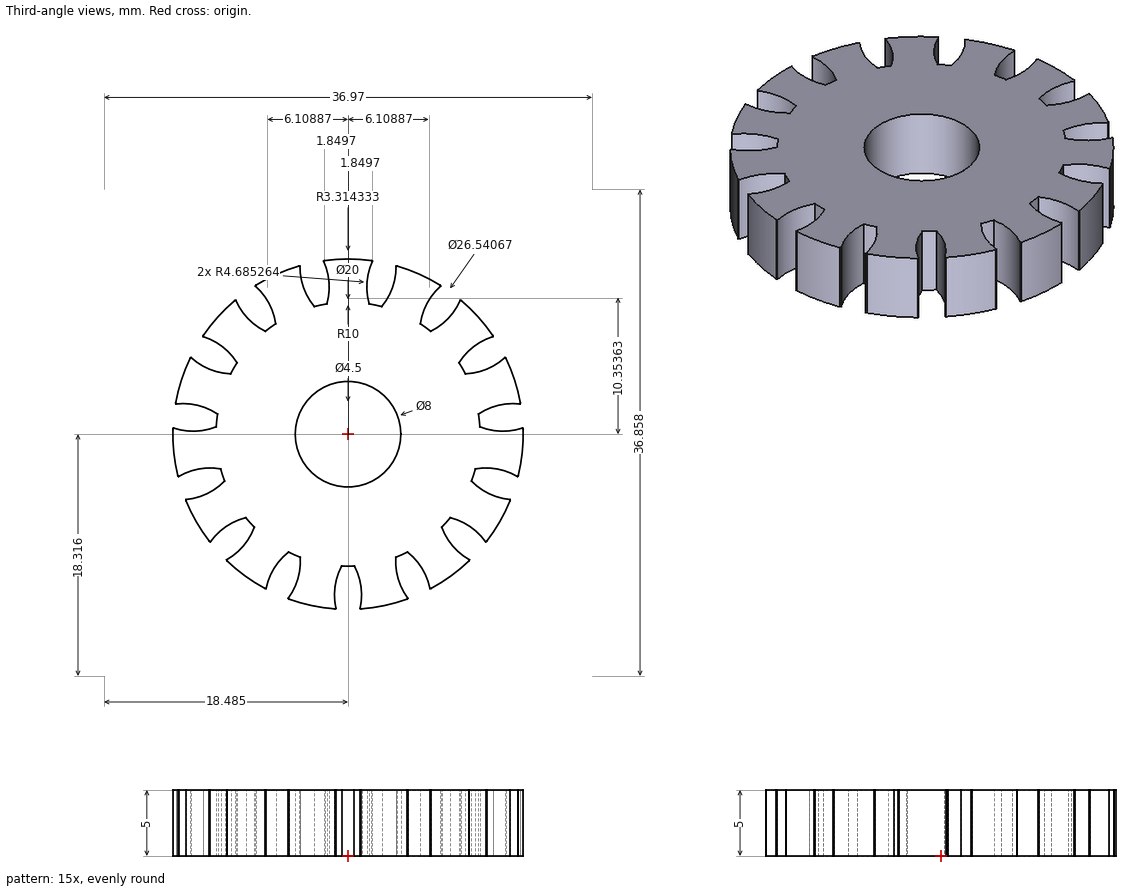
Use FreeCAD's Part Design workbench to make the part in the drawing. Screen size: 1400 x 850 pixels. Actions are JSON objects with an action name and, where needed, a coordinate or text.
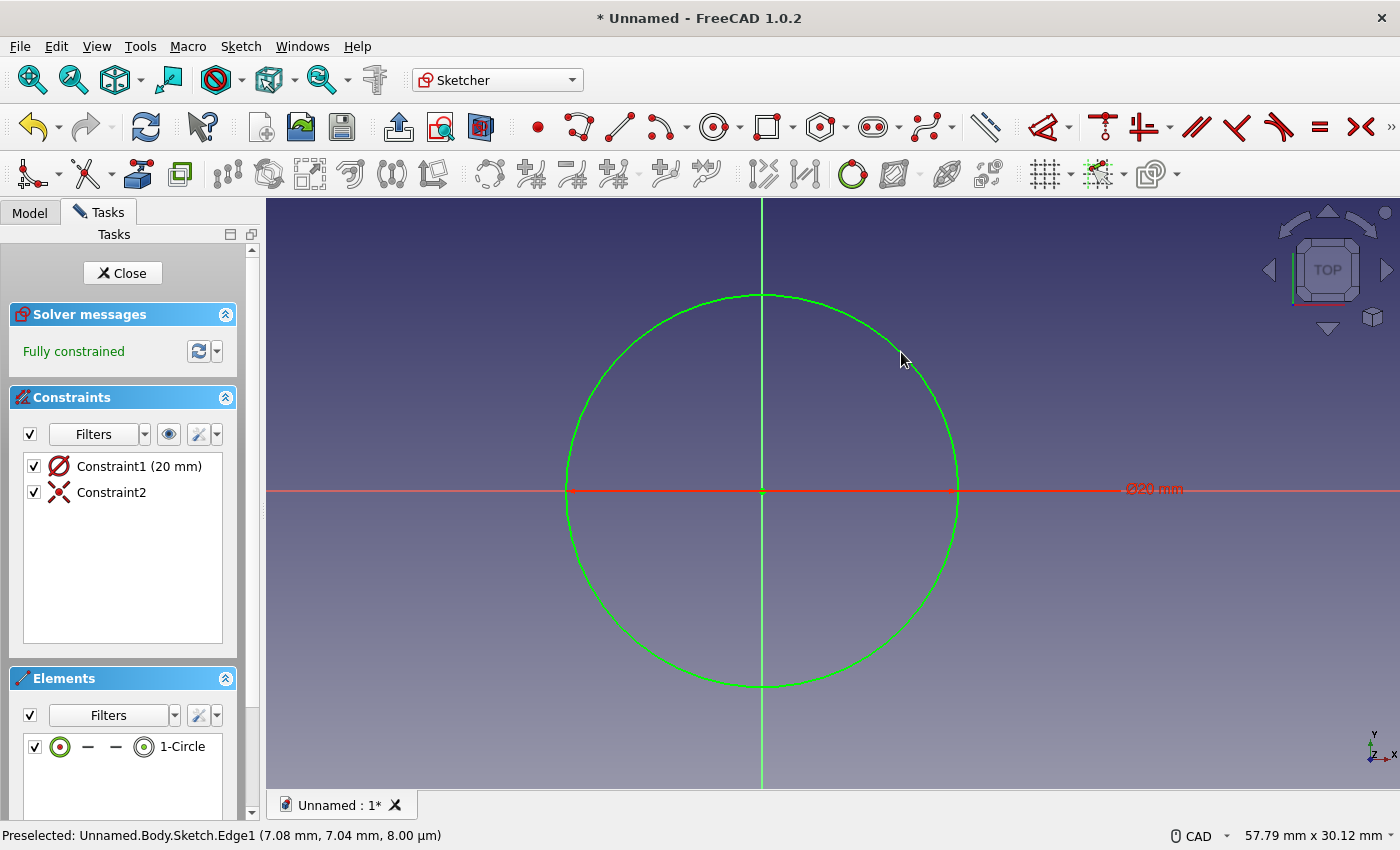
{"action": "left_click", "coordinate": [123, 273]}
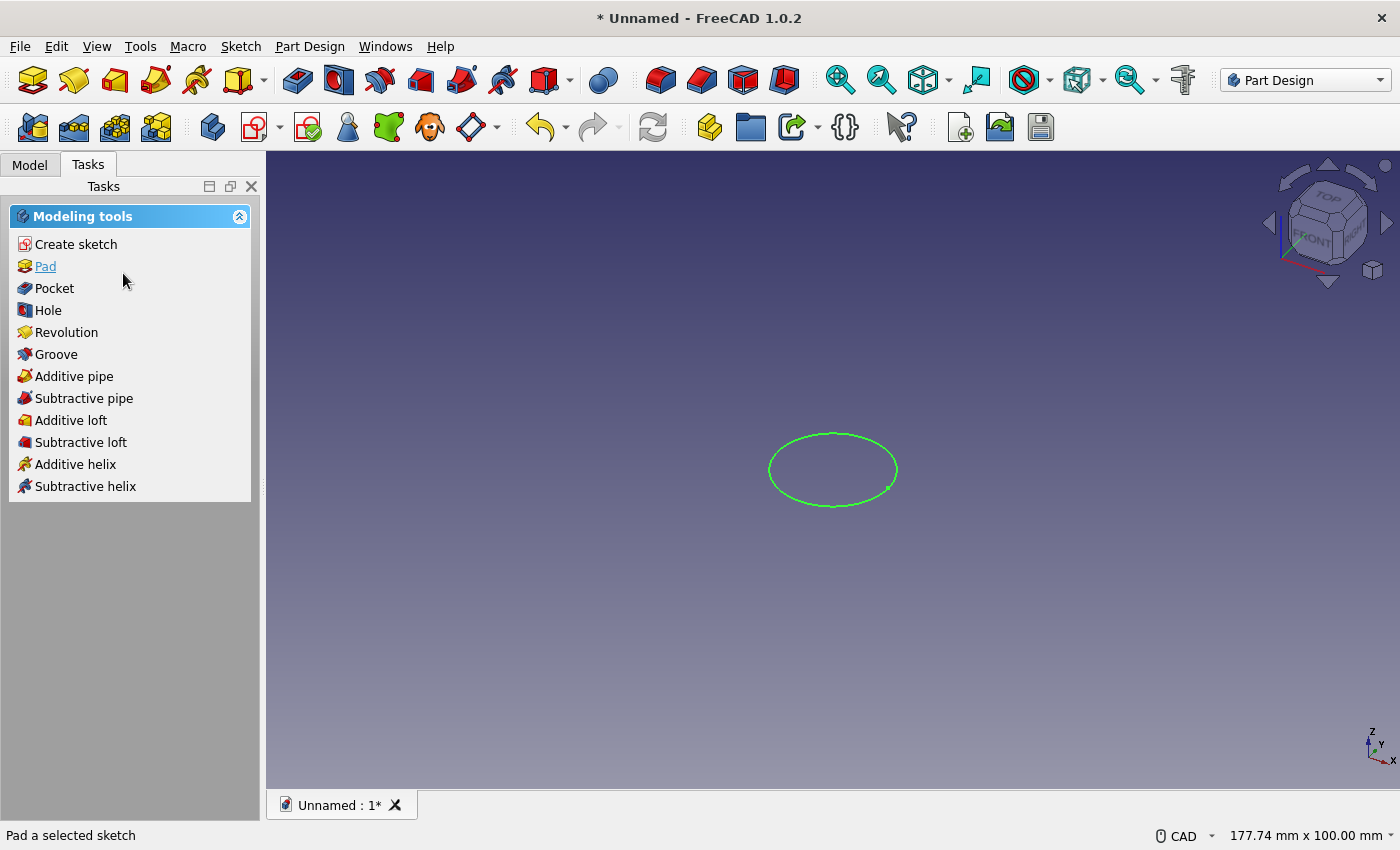
{"action": "left_click", "coordinate": [33, 80]}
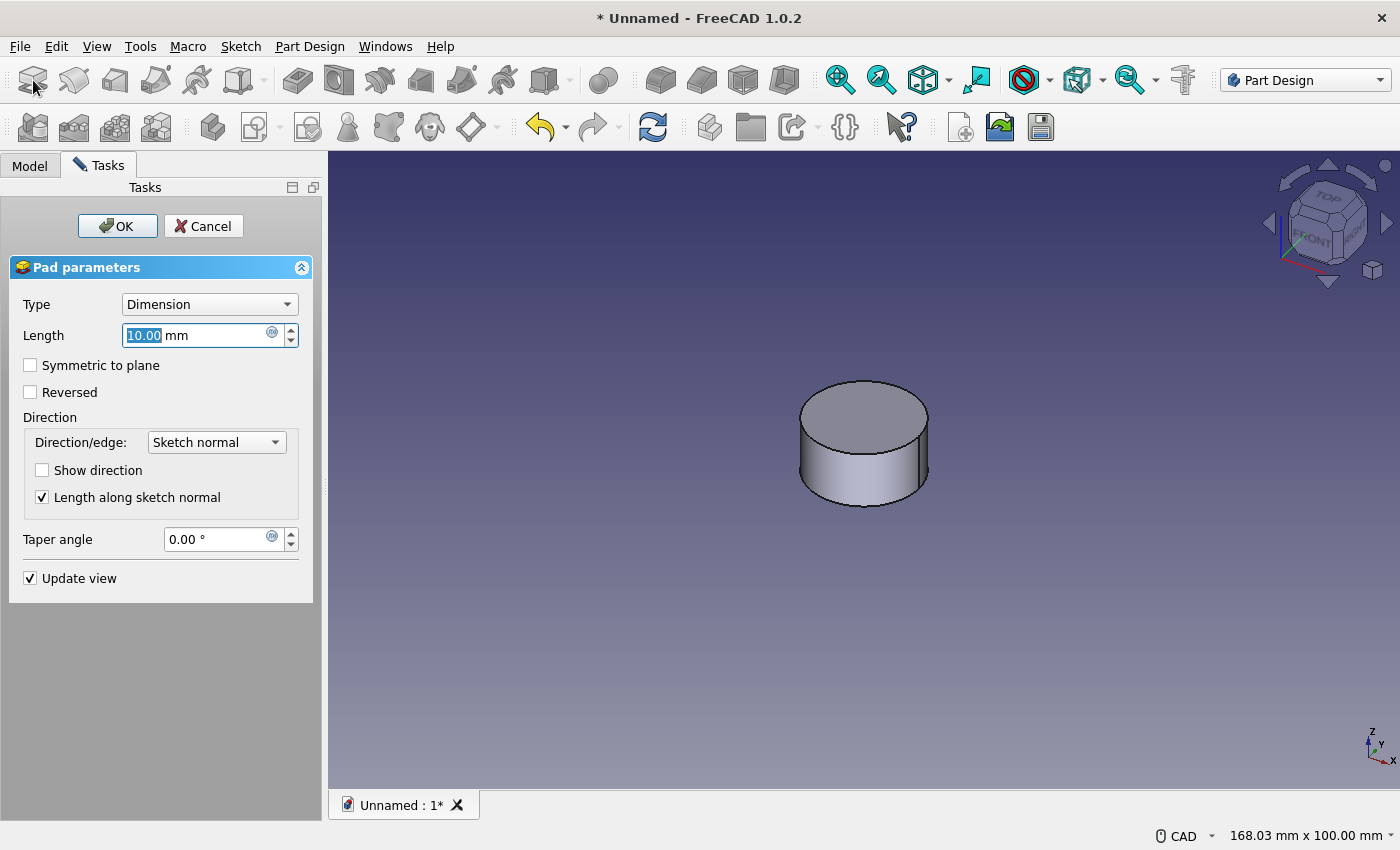
{"action": "type", "text": "5"}
{"action": "key", "text": "Tab"}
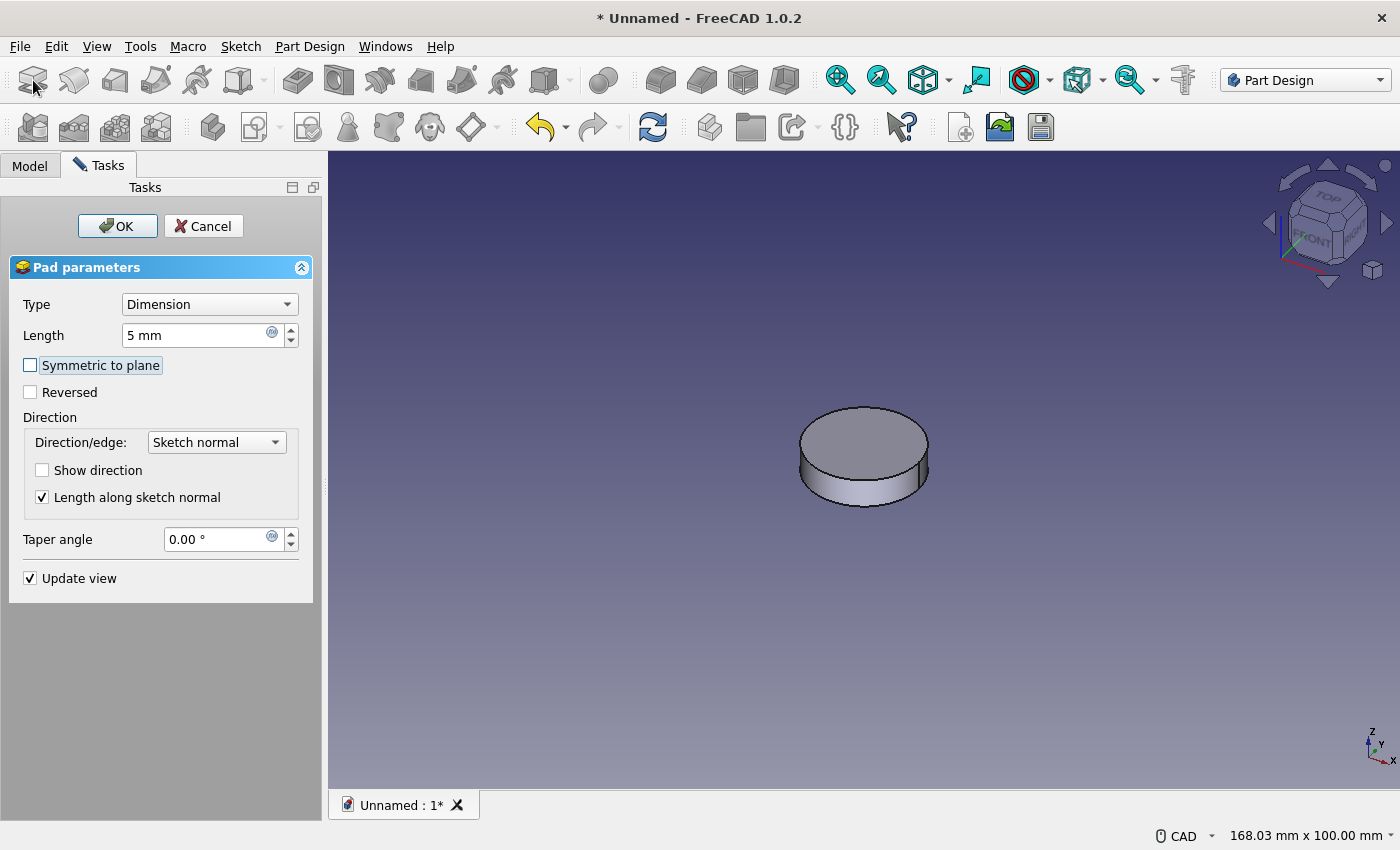
{"action": "left_click", "coordinate": [118, 226]}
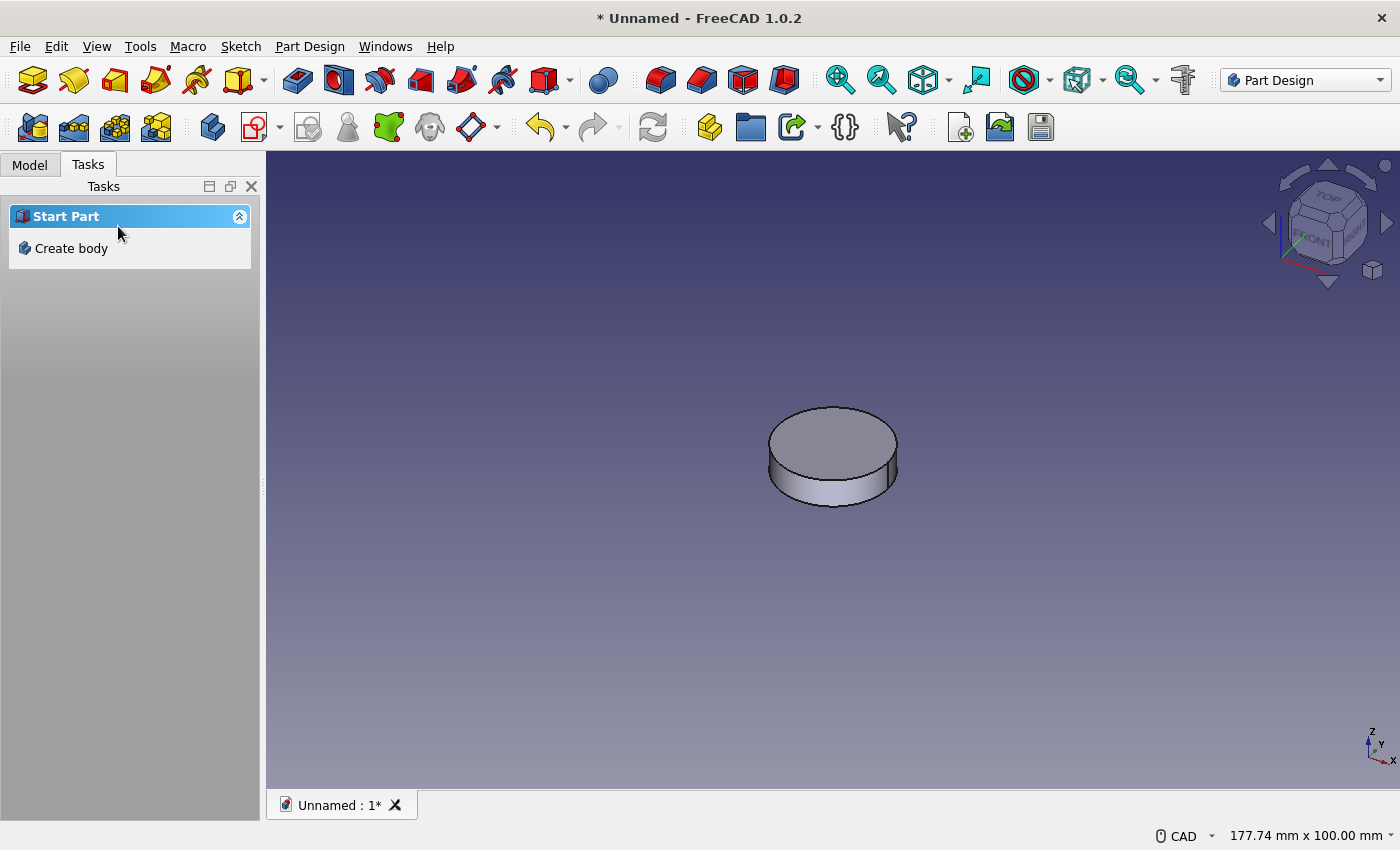
{"action": "key", "text": "v f"}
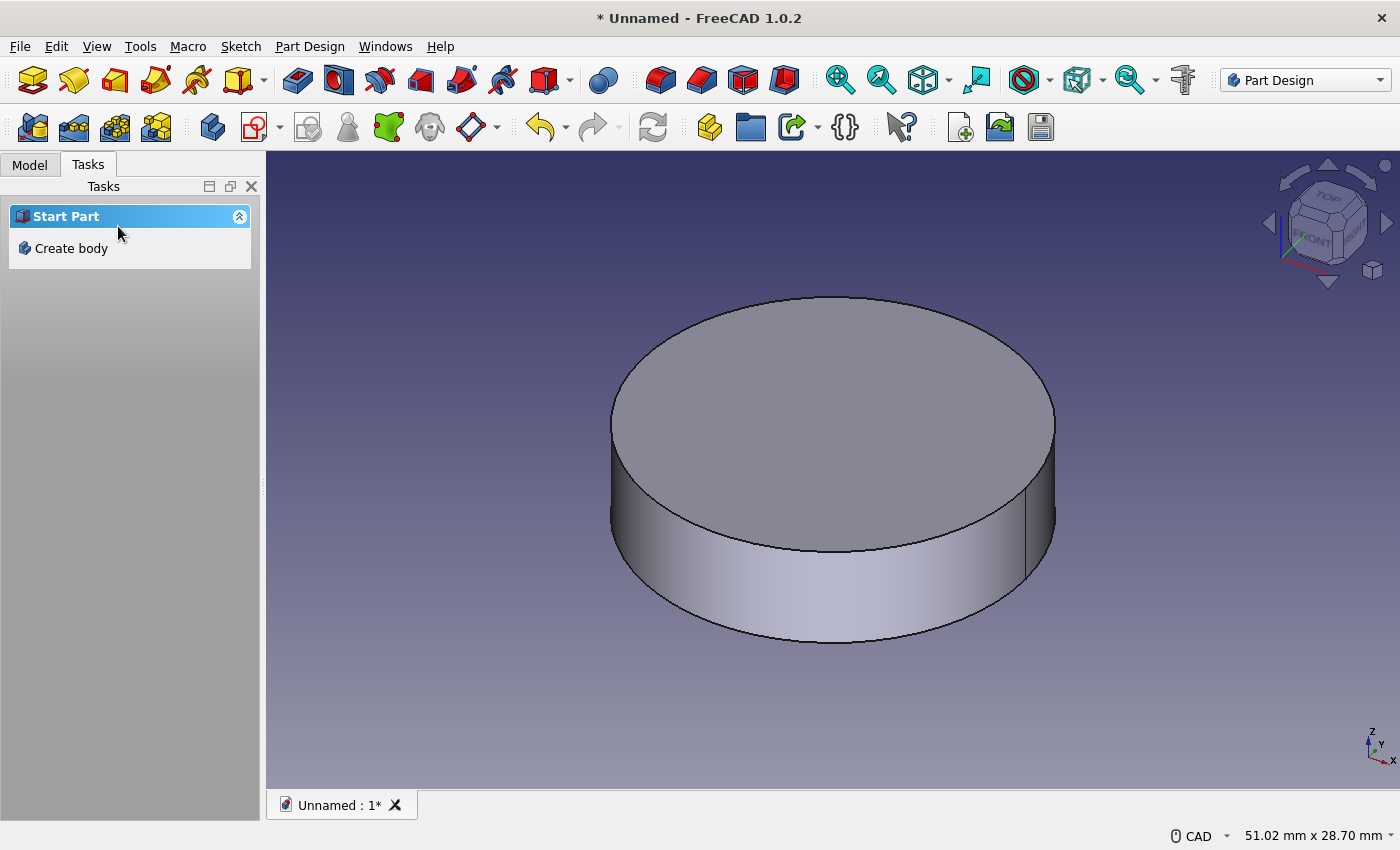
{"action": "left_click", "coordinate": [254, 128]}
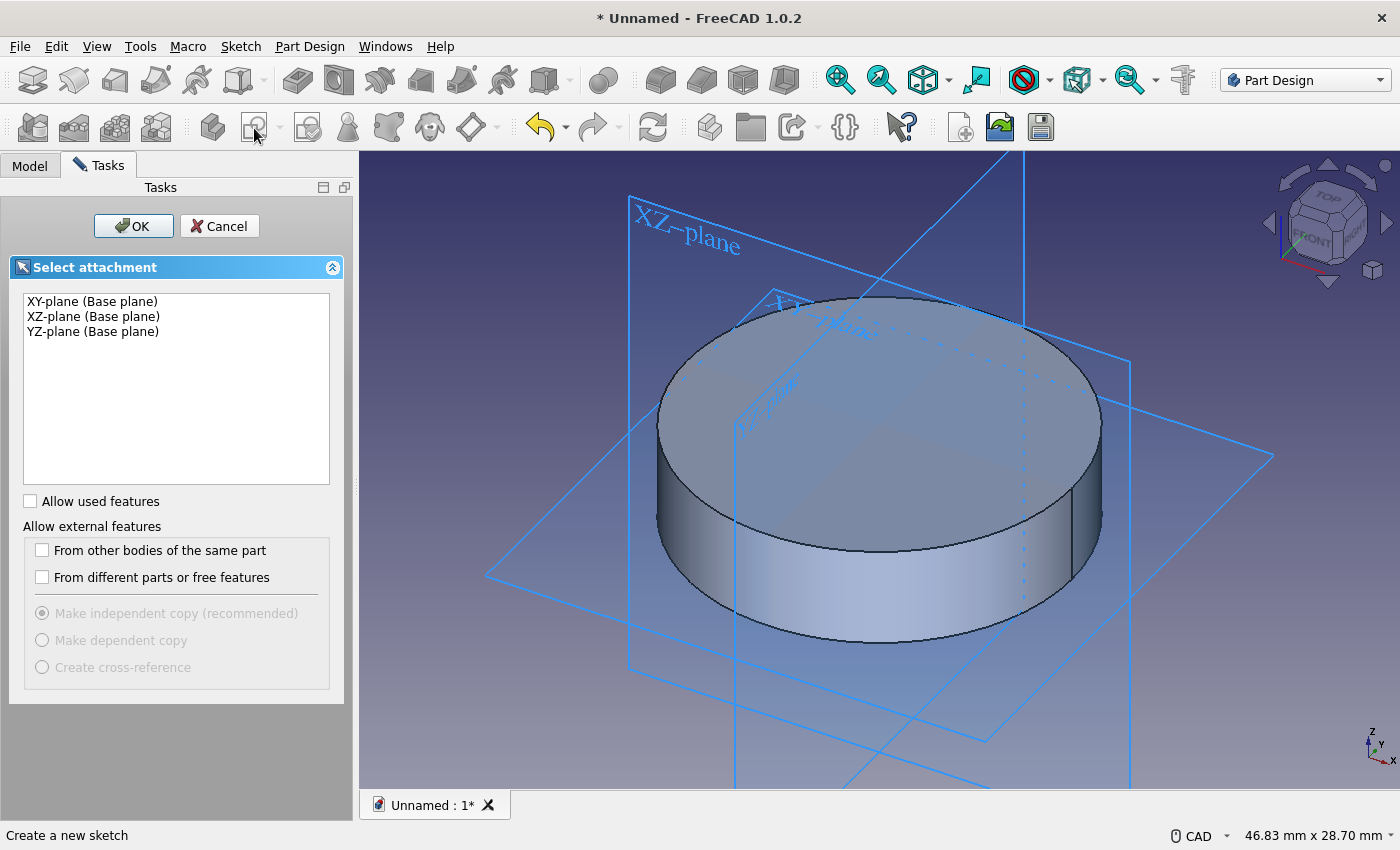
{"action": "left_click", "coordinate": [84, 302]}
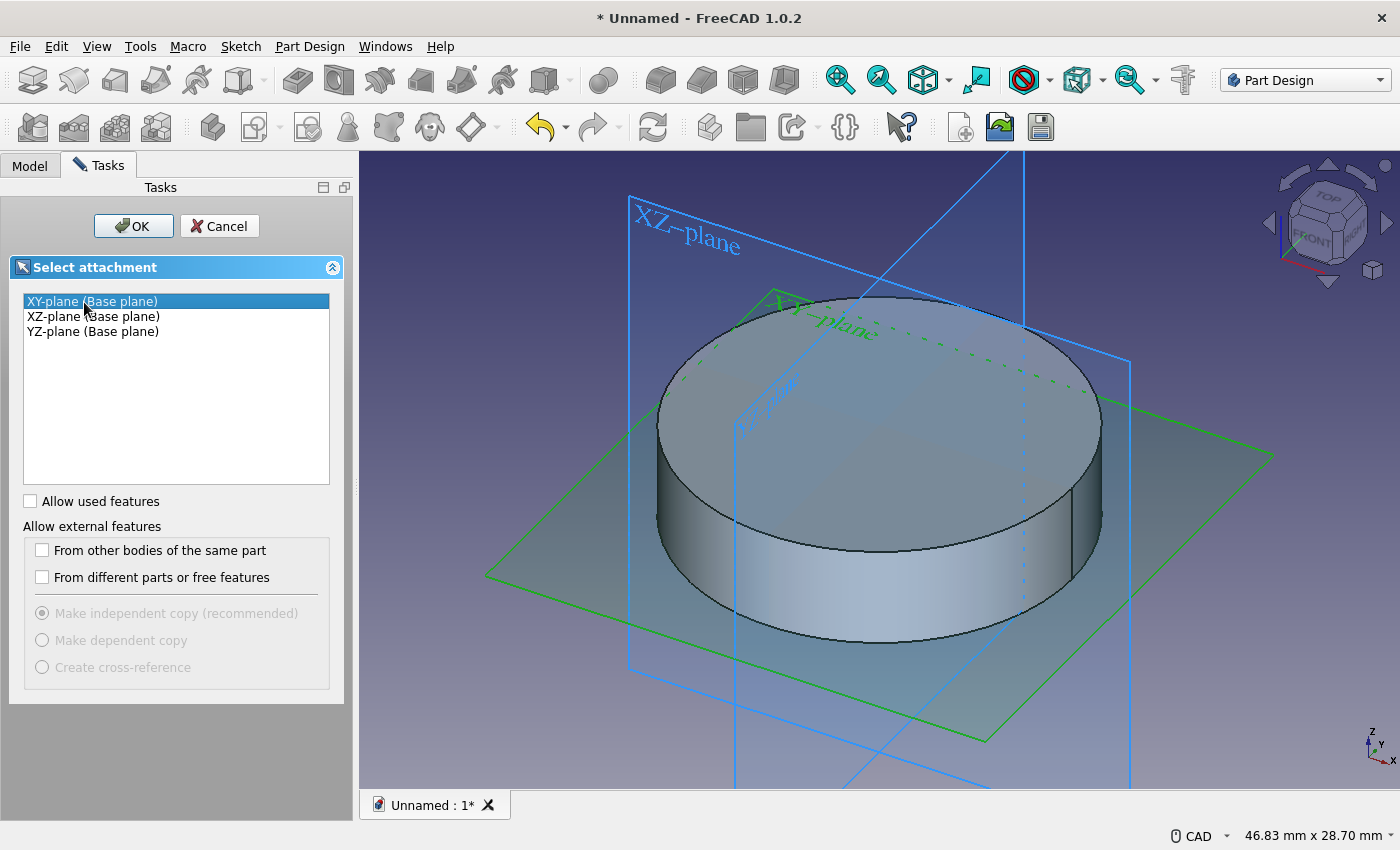
{"action": "left_click", "coordinate": [134, 226]}